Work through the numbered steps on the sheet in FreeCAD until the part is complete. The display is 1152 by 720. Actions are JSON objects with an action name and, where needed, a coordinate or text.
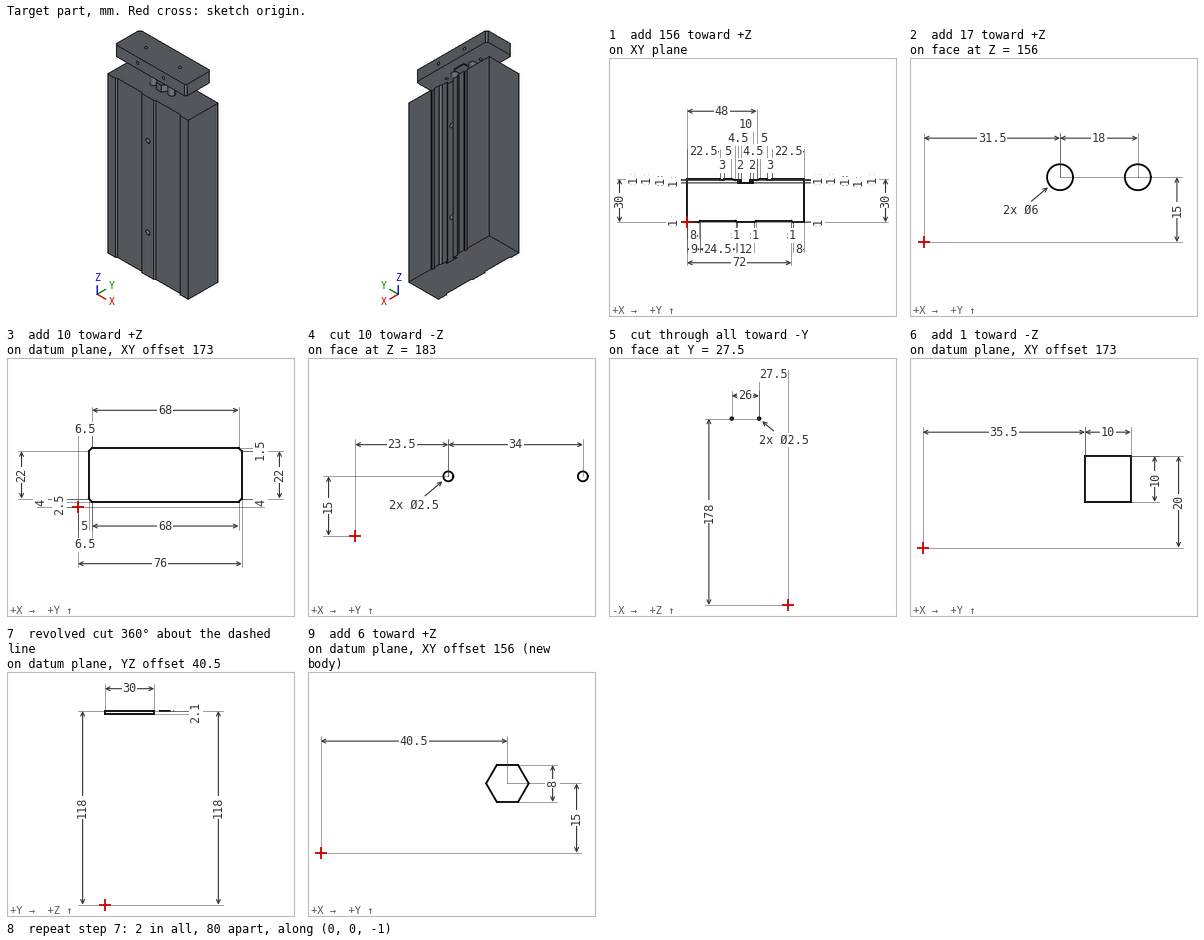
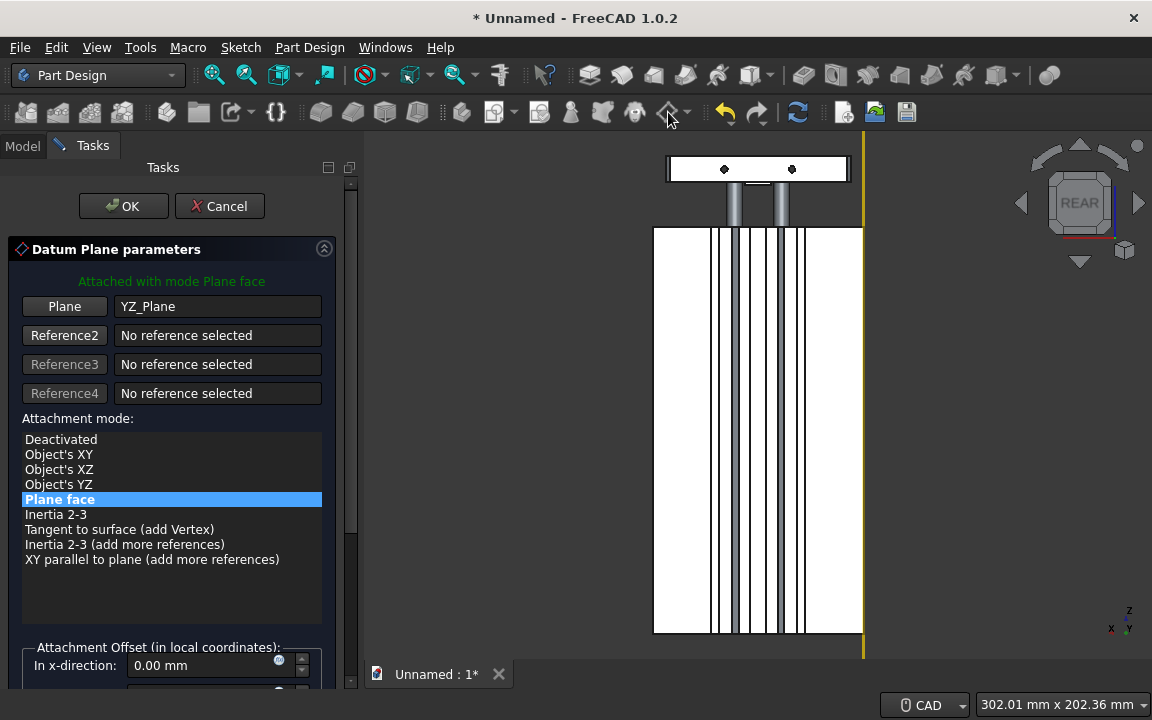
{"action": "scroll", "coordinate": [351, 432], "scroll_direction": "down", "scroll_amount": 2}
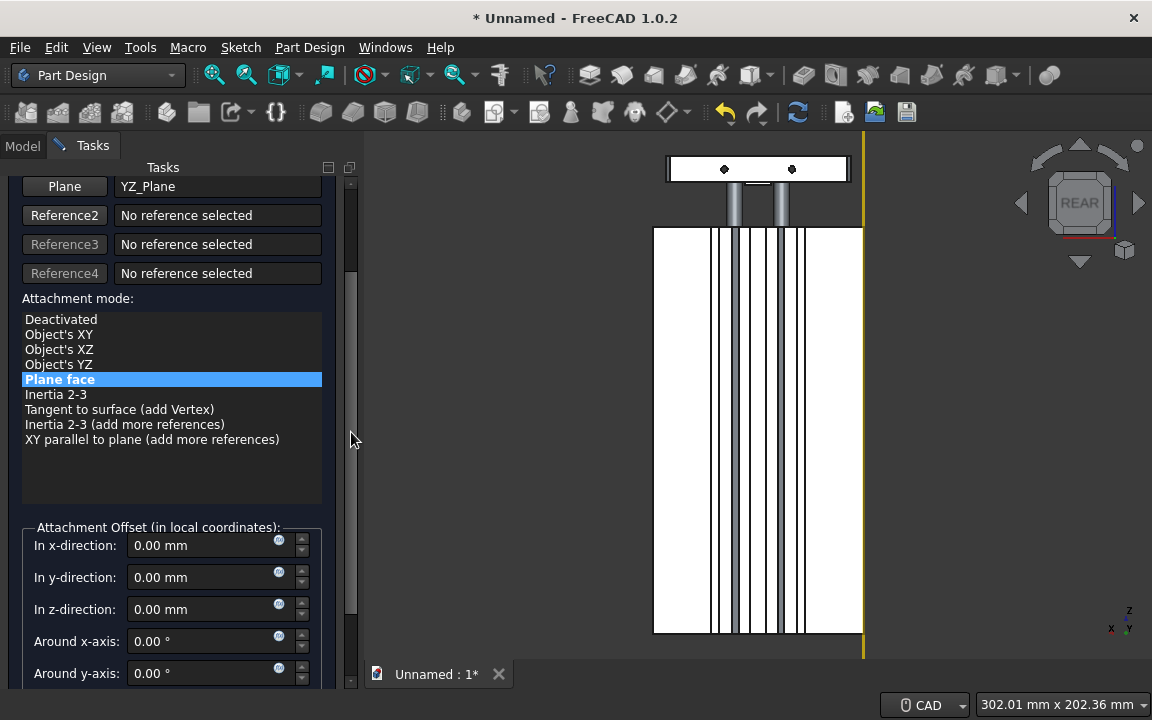
{"action": "triple_click", "coordinate": [210, 609]}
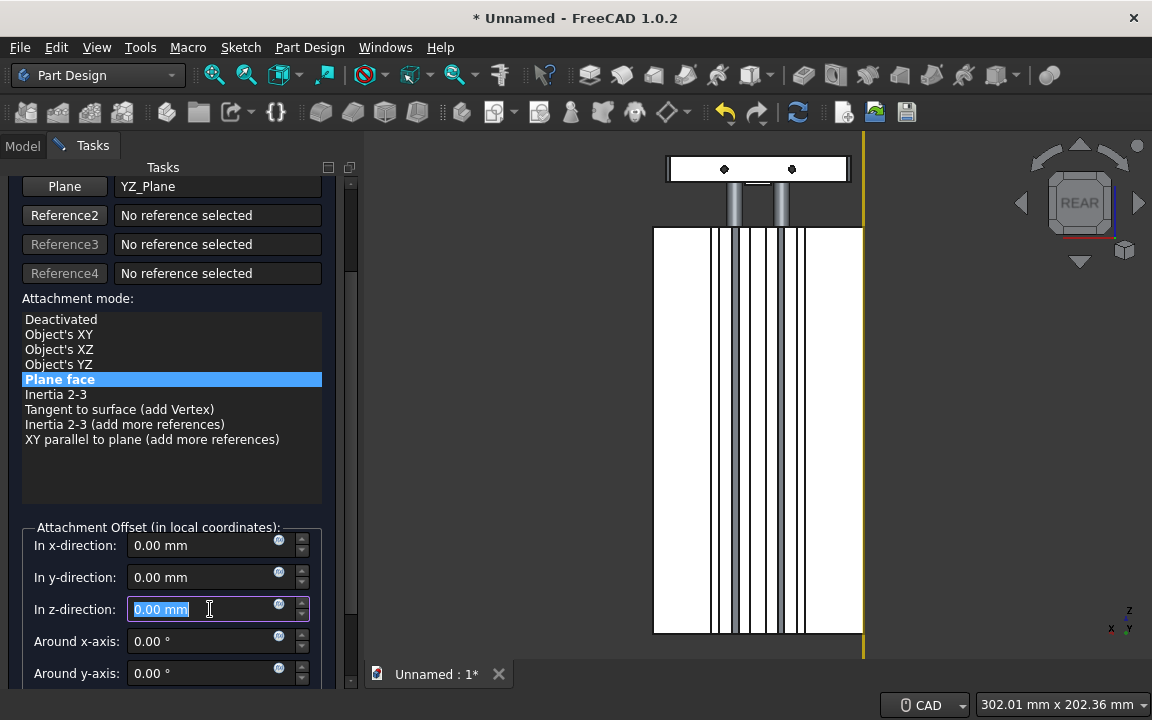
{"action": "type", "text": "40.5"}
{"action": "key", "text": "Tab"}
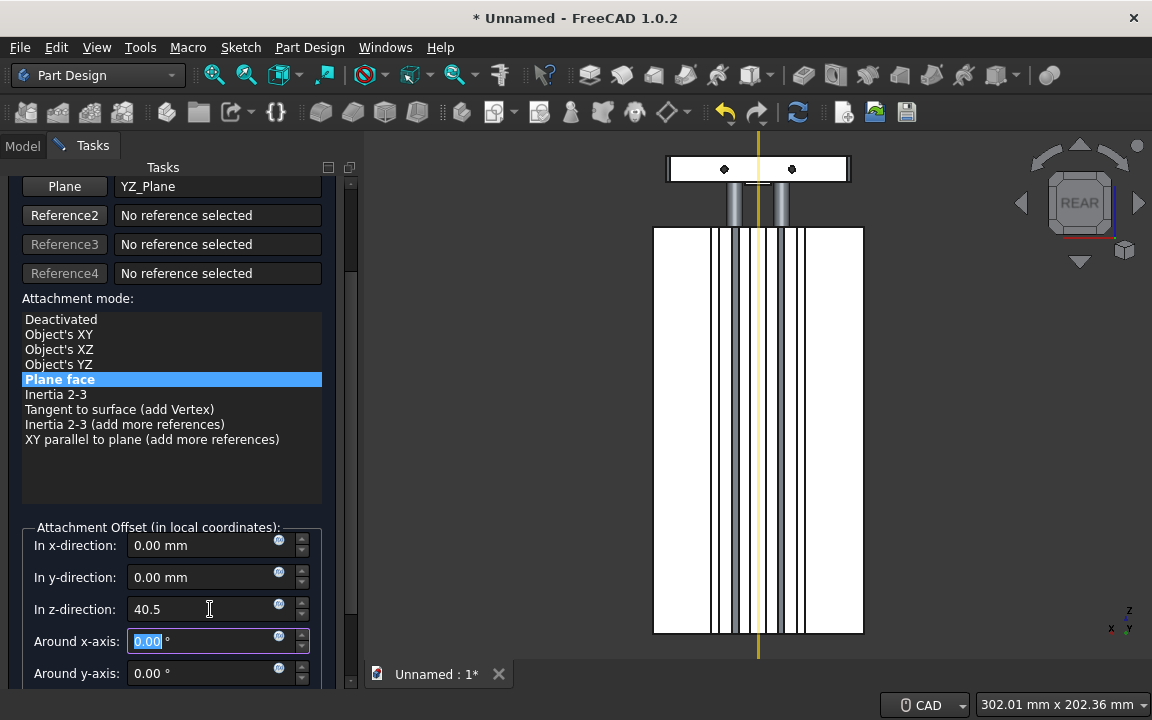
{"action": "scroll", "coordinate": [351, 432], "scroll_direction": "up", "scroll_amount": 3}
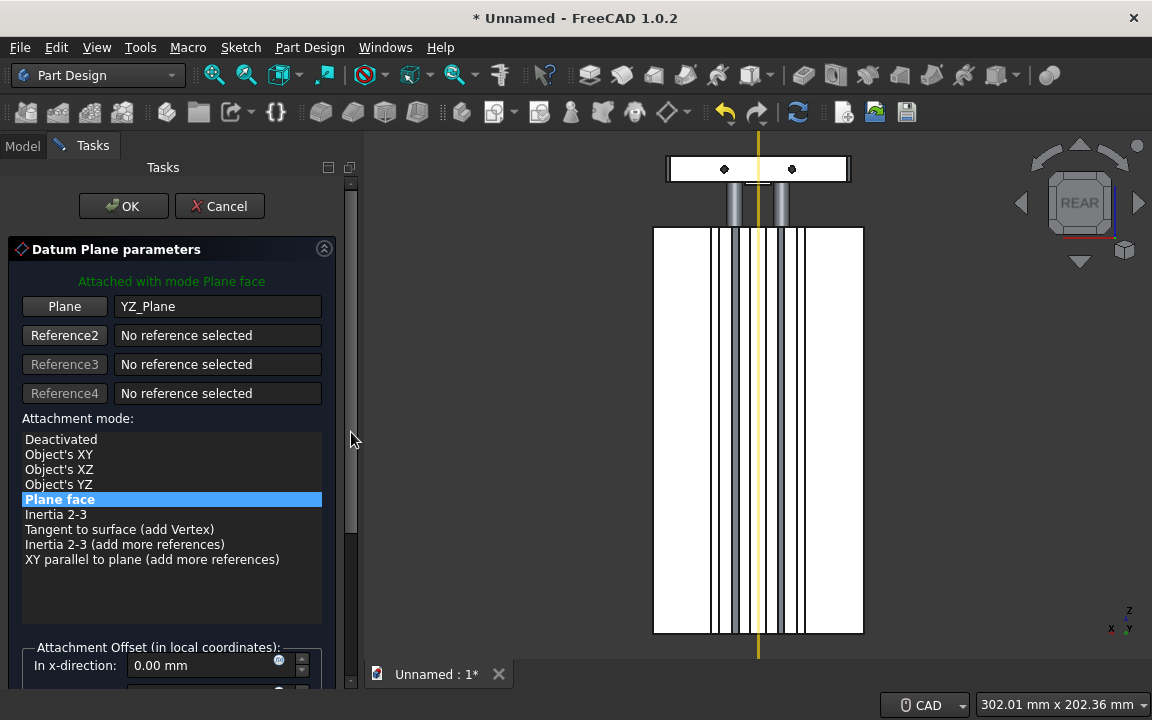
{"action": "left_click", "coordinate": [124, 206]}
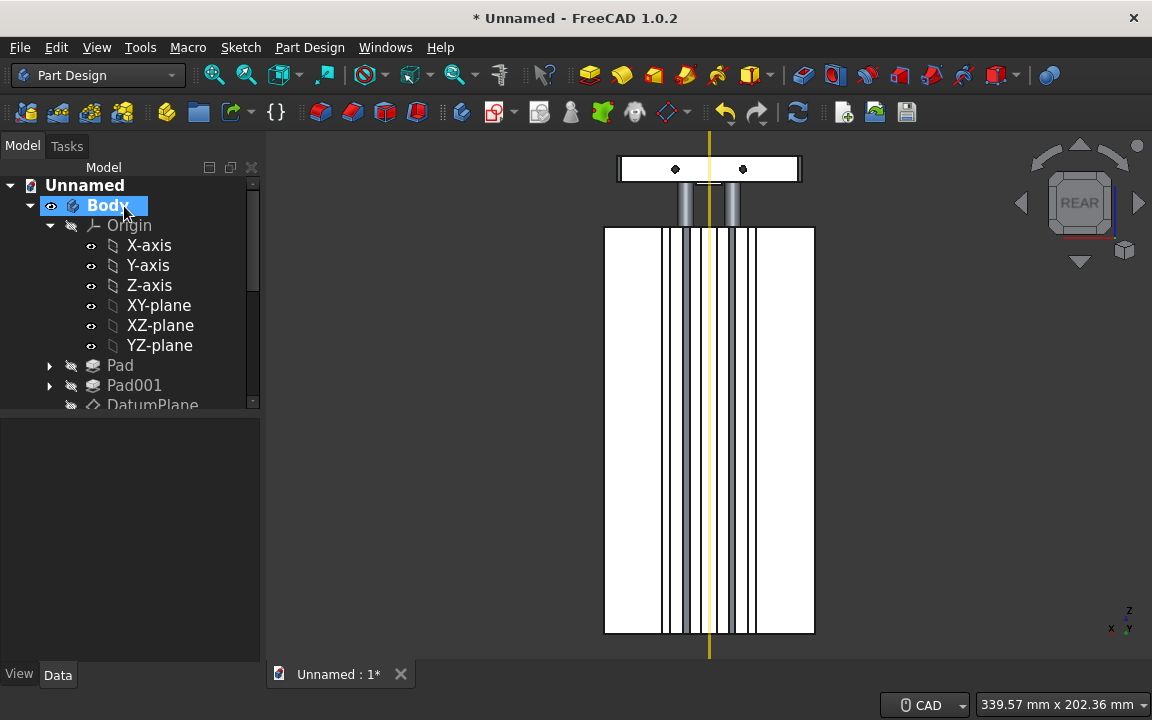
{"action": "scroll", "coordinate": [100, 301], "scroll_direction": "down", "scroll_amount": 3}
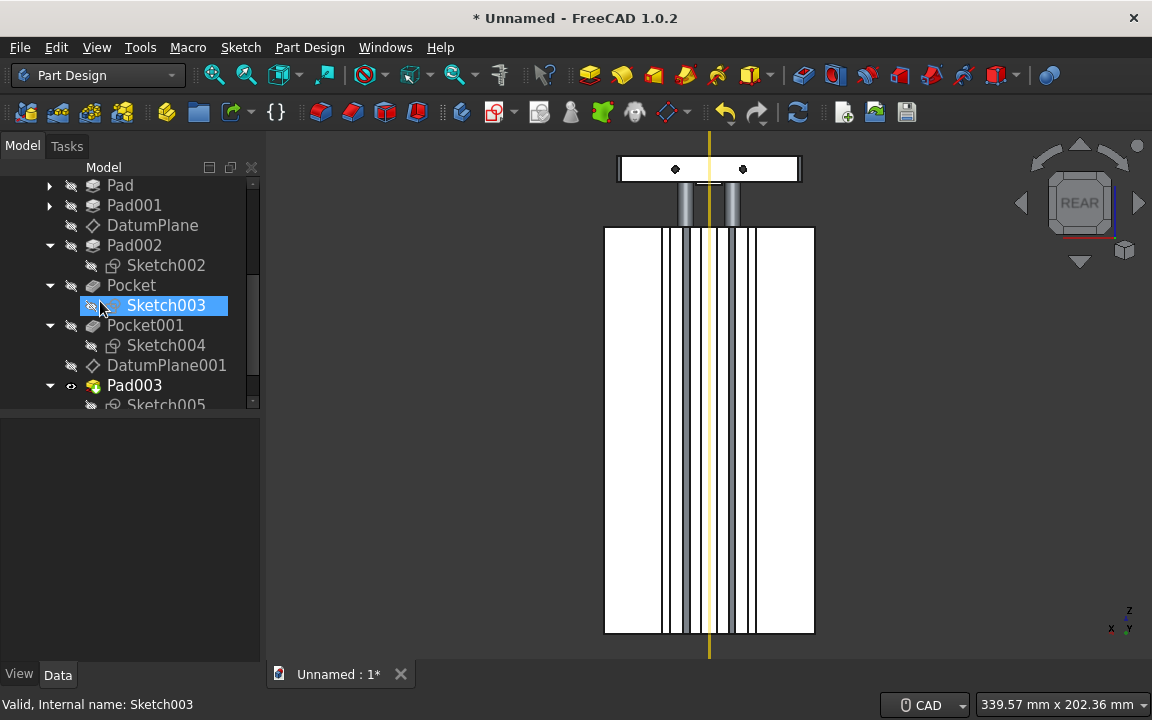
{"action": "scroll", "coordinate": [140, 301], "scroll_direction": "up", "scroll_amount": 15}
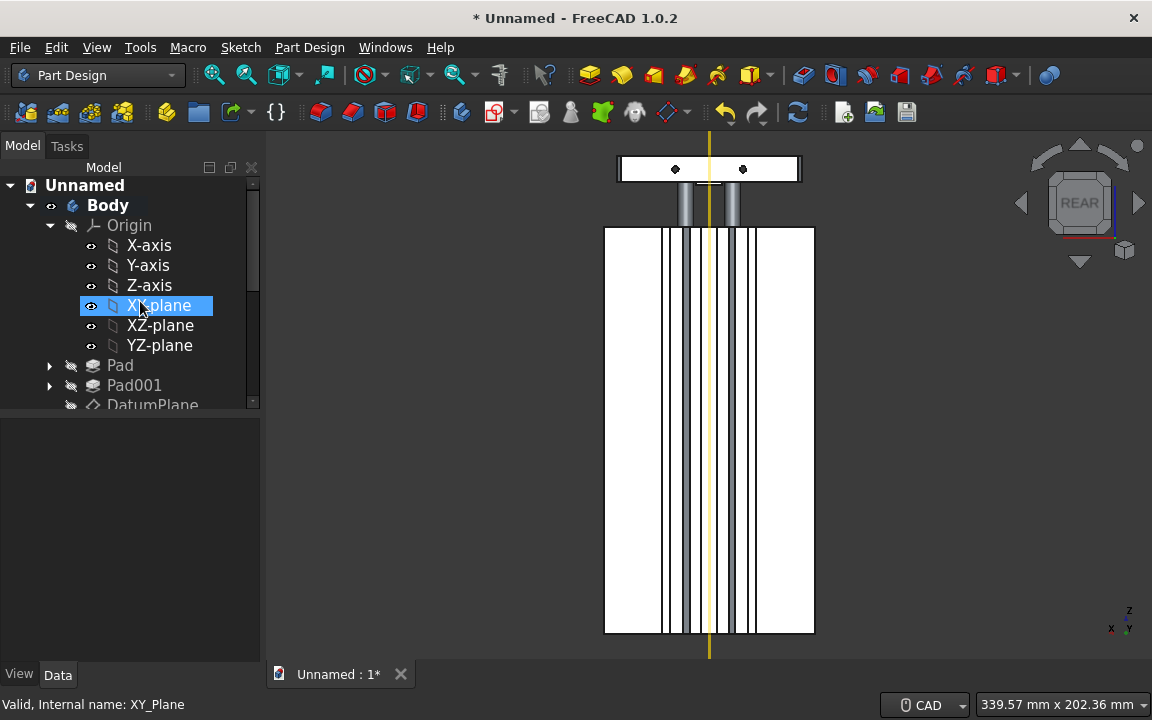
{"action": "scroll", "coordinate": [100, 301], "scroll_direction": "down", "scroll_amount": 6}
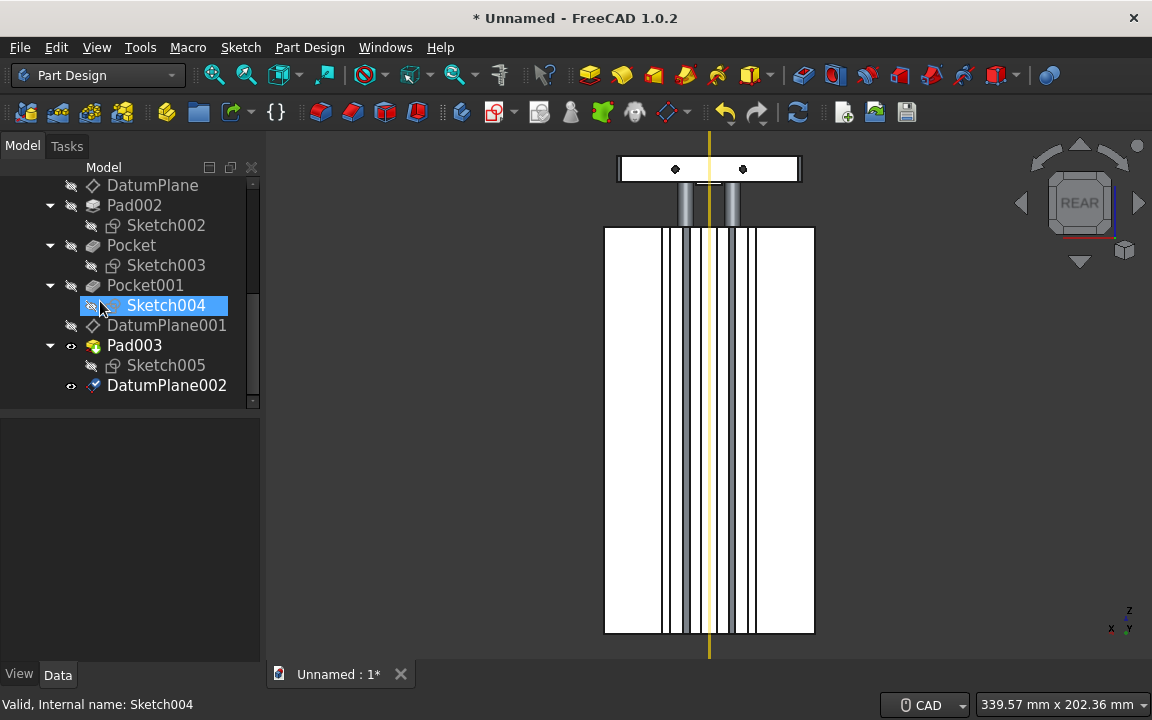
{"action": "left_click", "coordinate": [116, 386]}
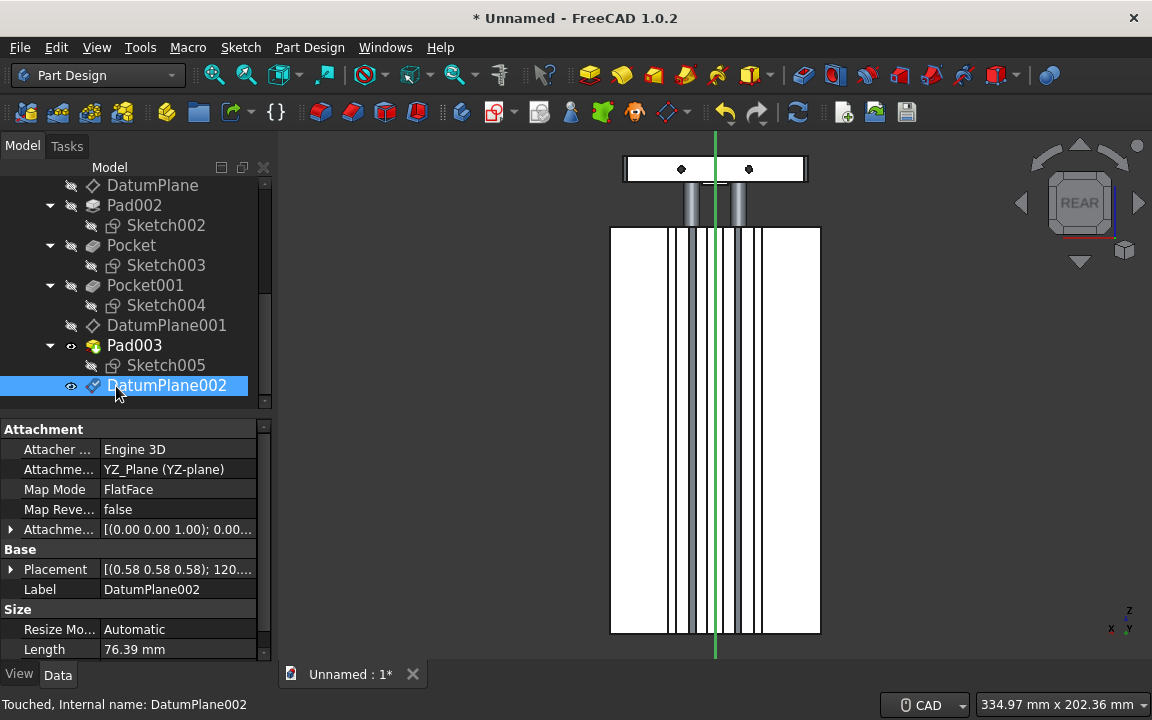
{"action": "left_click", "coordinate": [494, 112]}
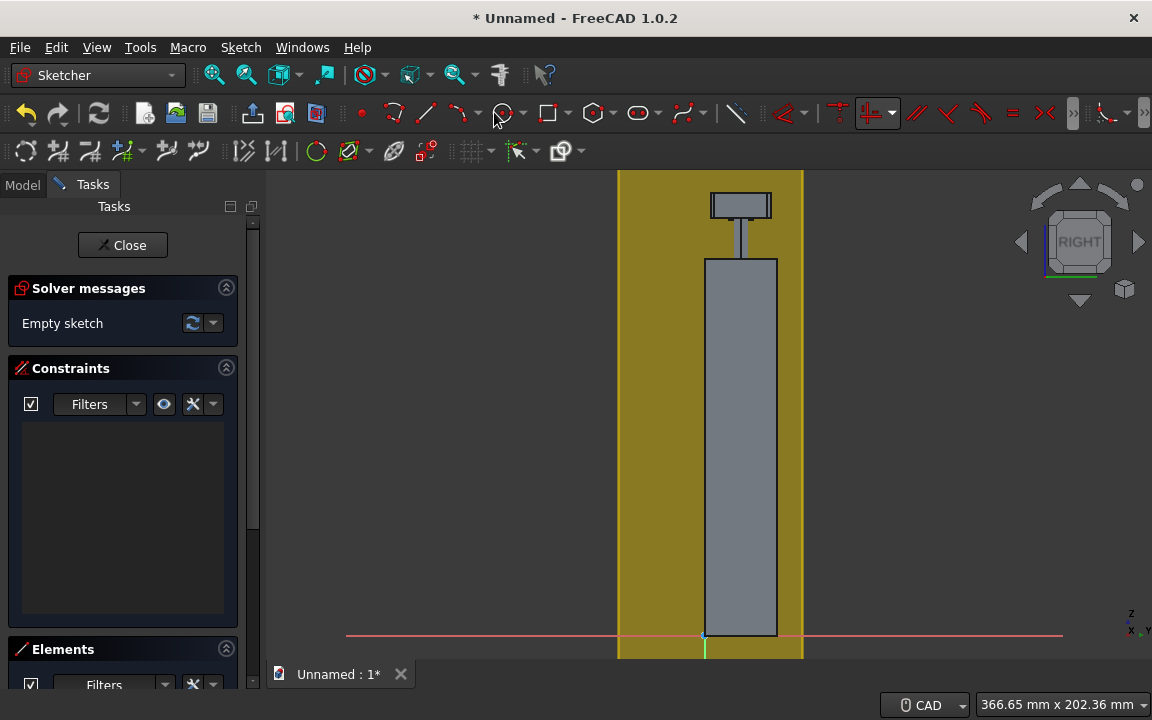
{"action": "left_click", "coordinate": [318, 114]}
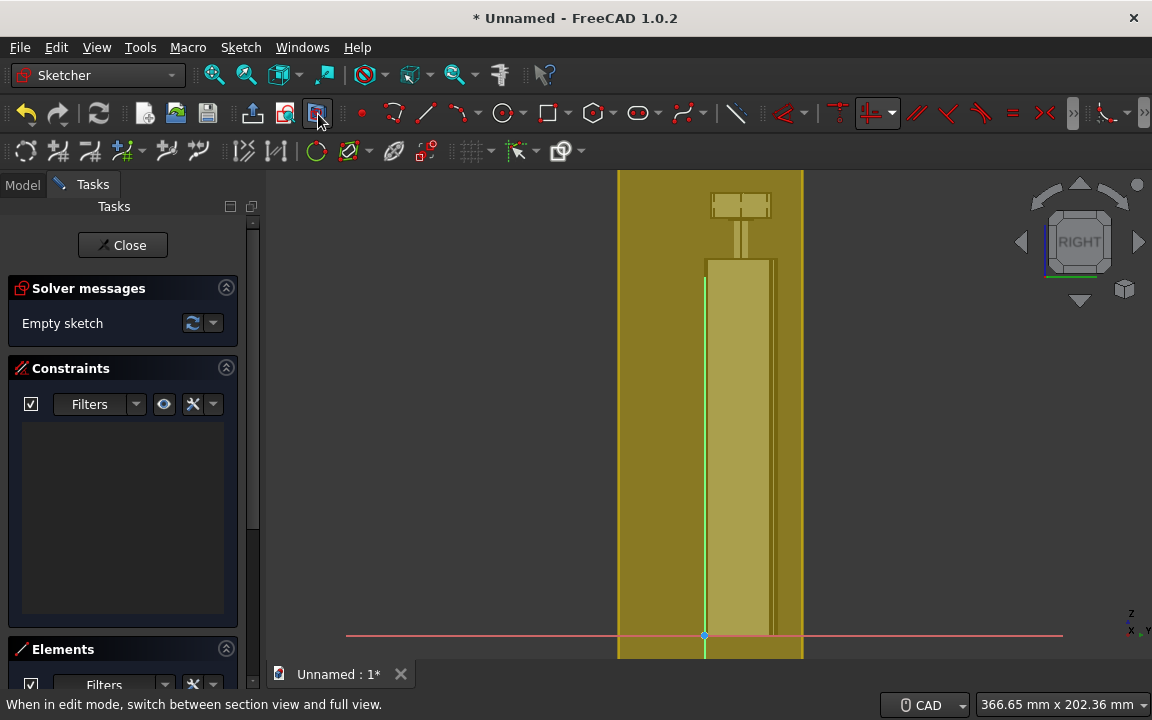
{"action": "scroll", "coordinate": [784, 337], "scroll_direction": "up", "scroll_amount": 8}